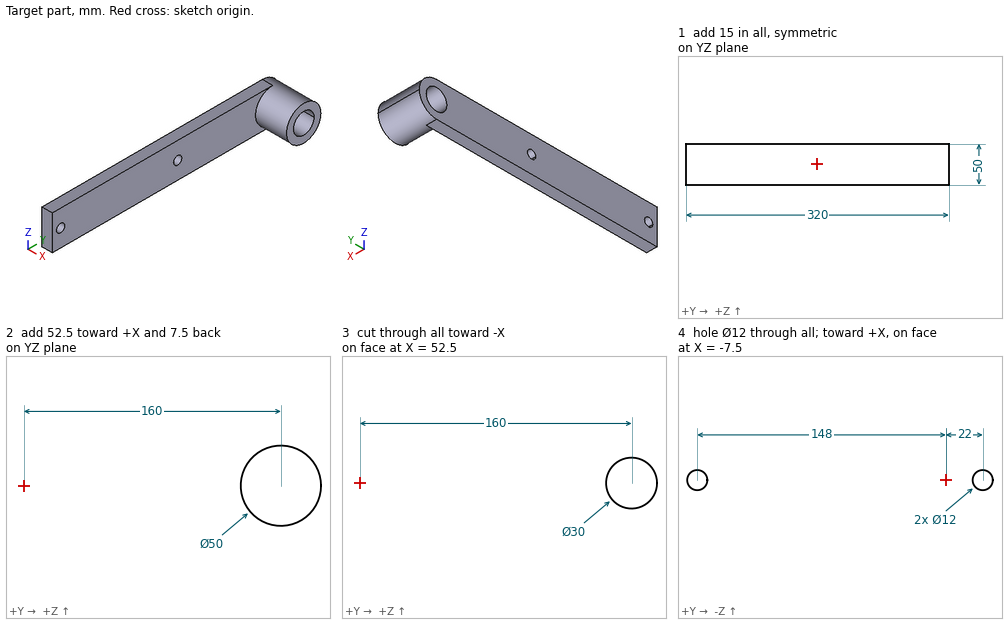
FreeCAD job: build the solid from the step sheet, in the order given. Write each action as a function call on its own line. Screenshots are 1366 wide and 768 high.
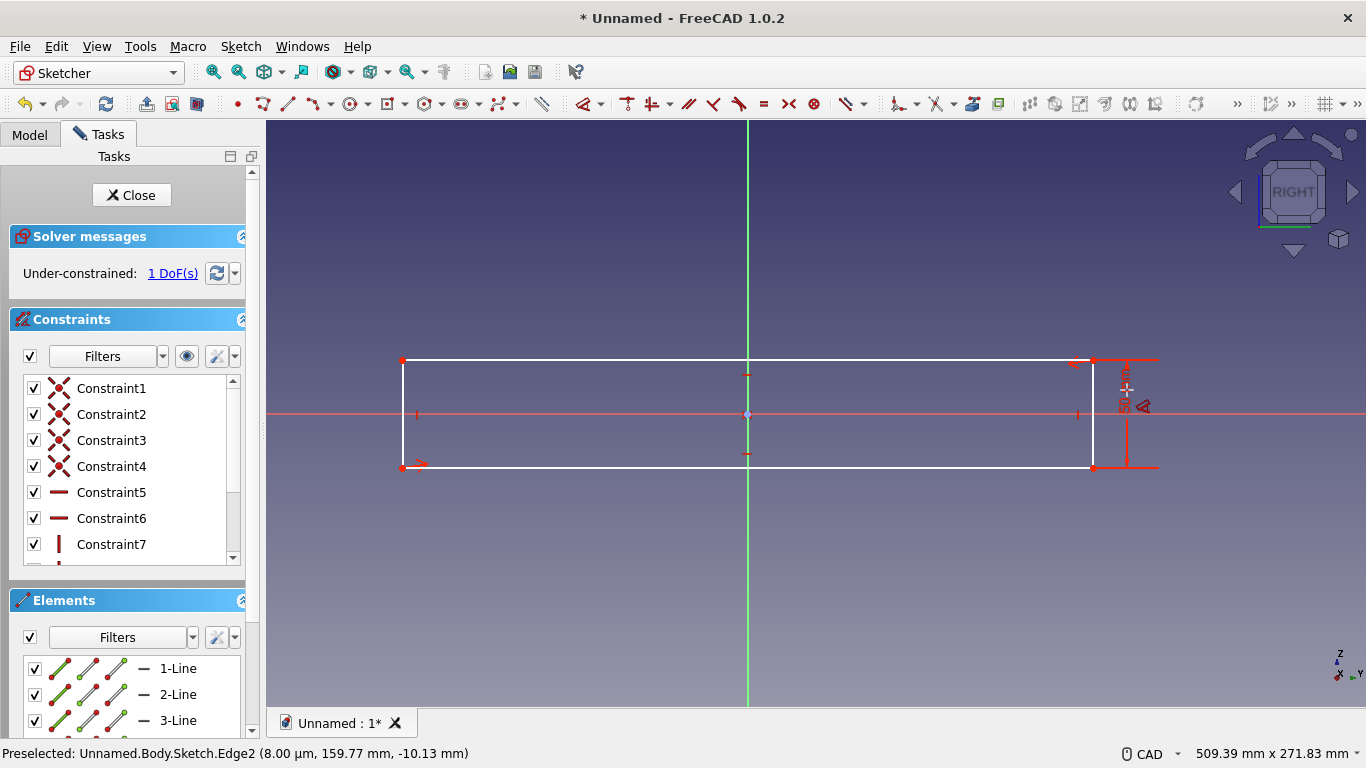
click(610, 468)
click(589, 502)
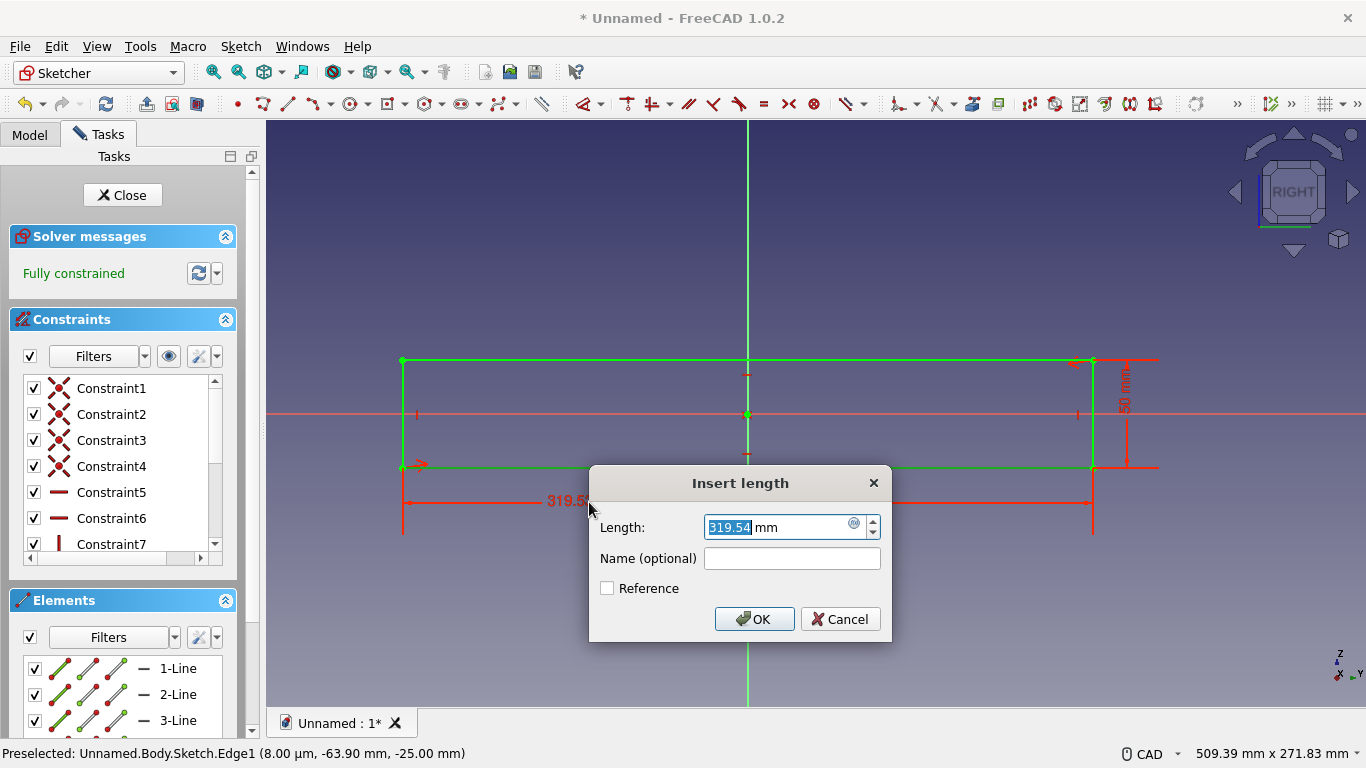
text(320)
key(Return)
key(Escape)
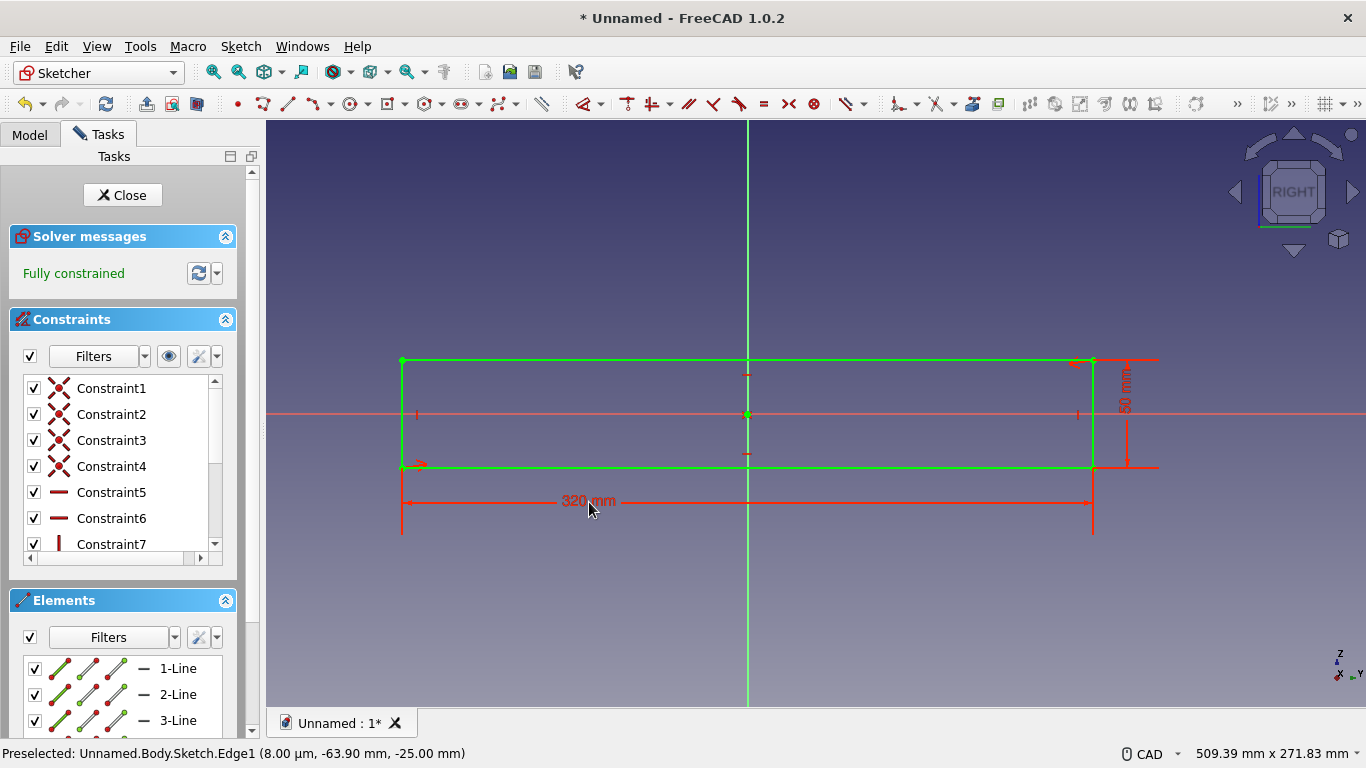
click(123, 195)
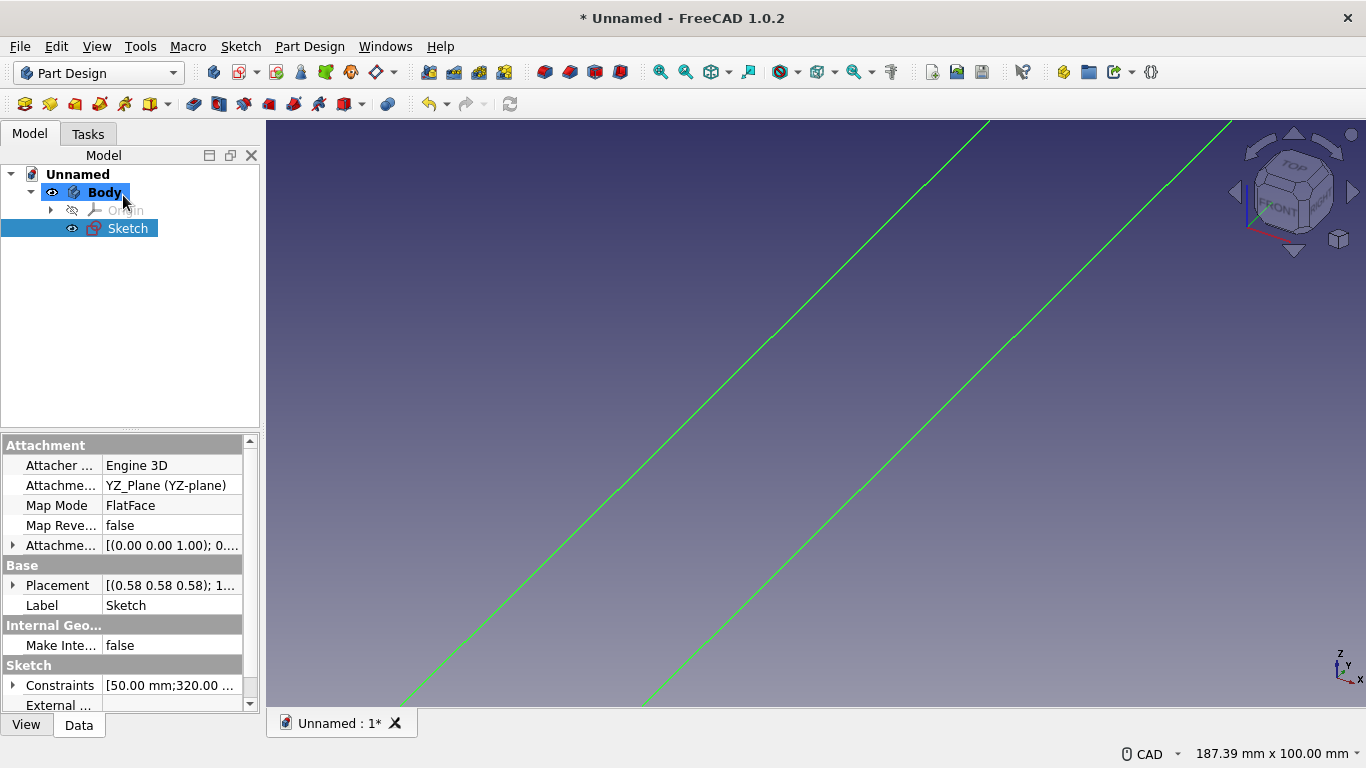
click(25, 104)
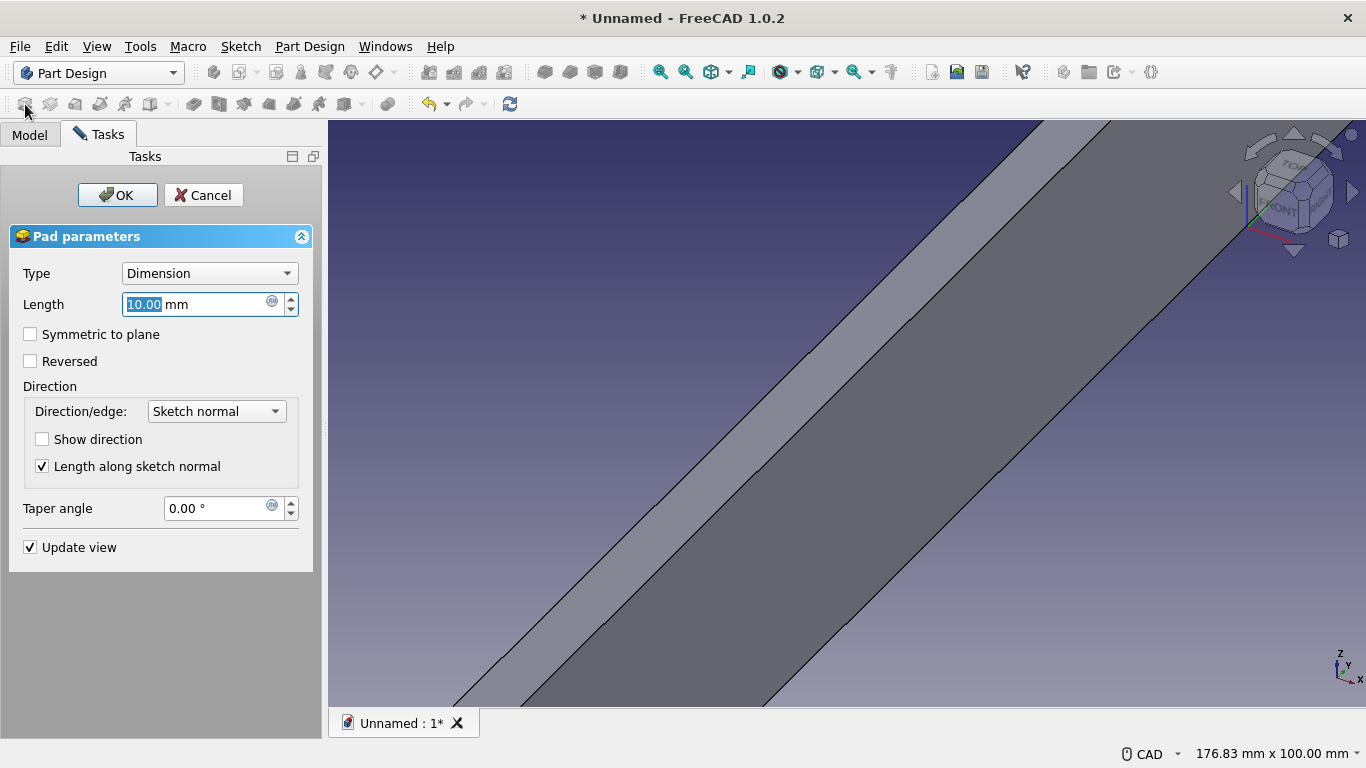
text(15)
key(Tab)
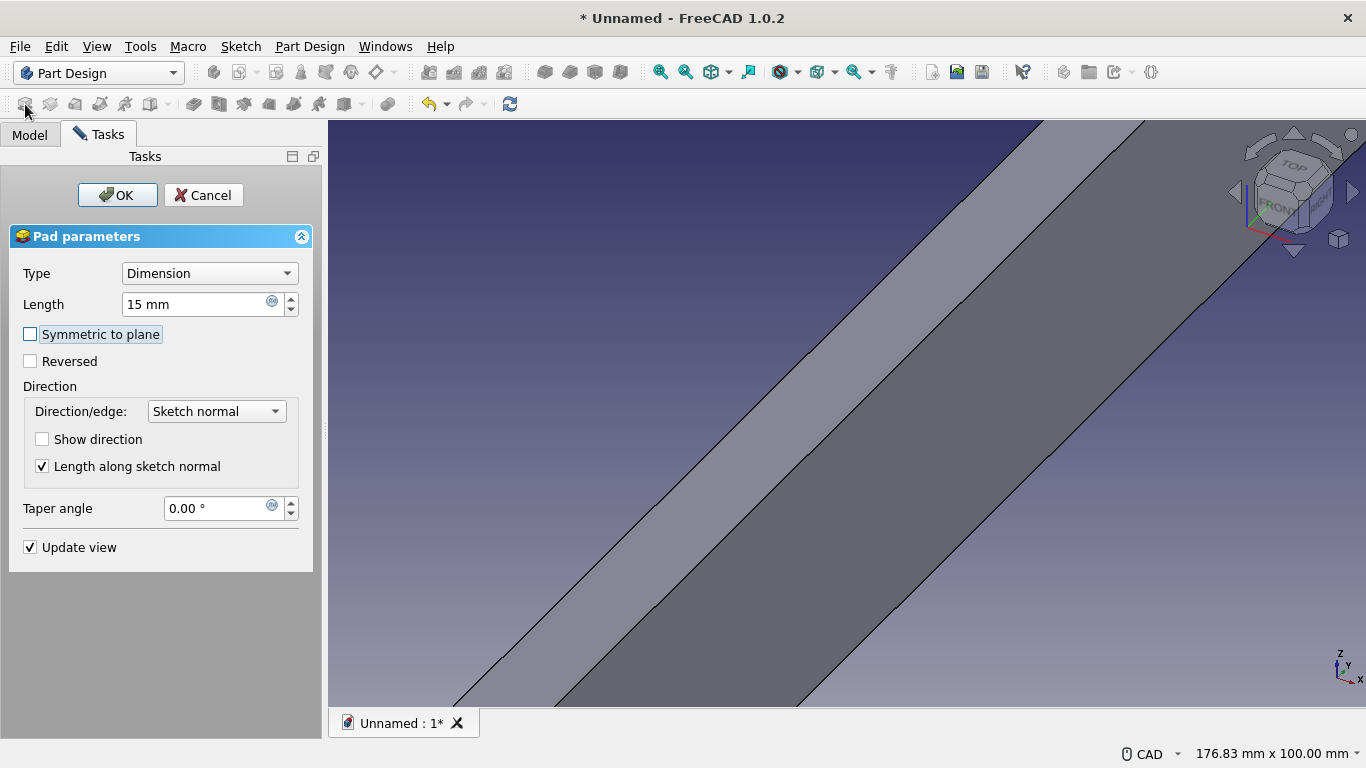
click(31, 334)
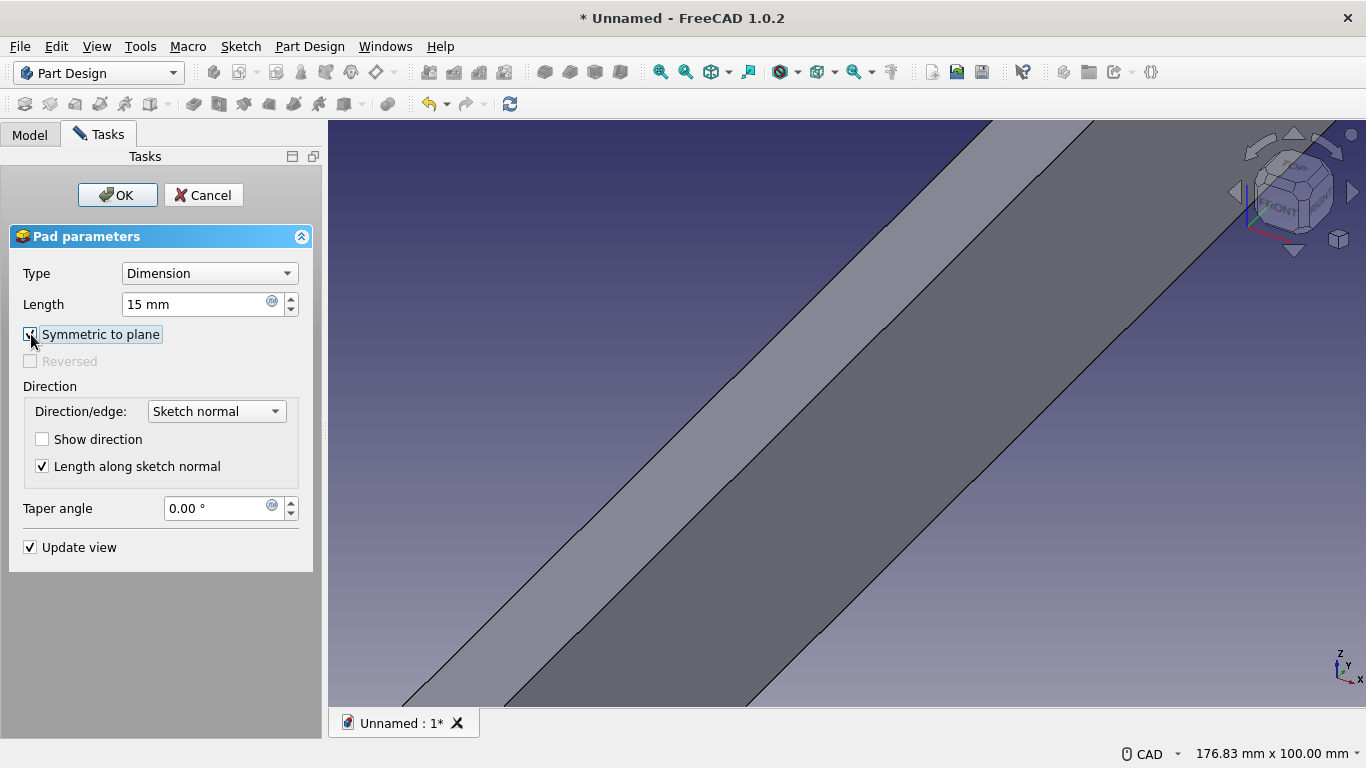
click(118, 195)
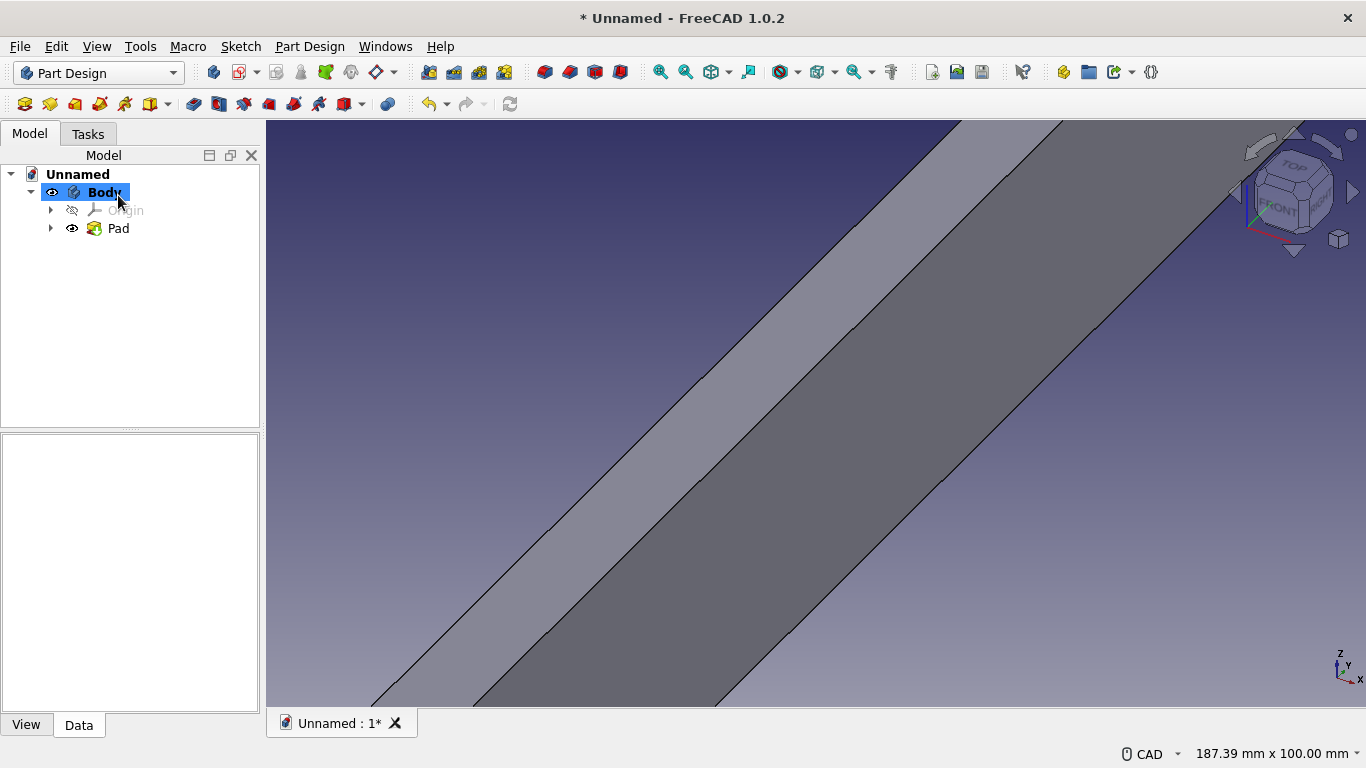
click(661, 72)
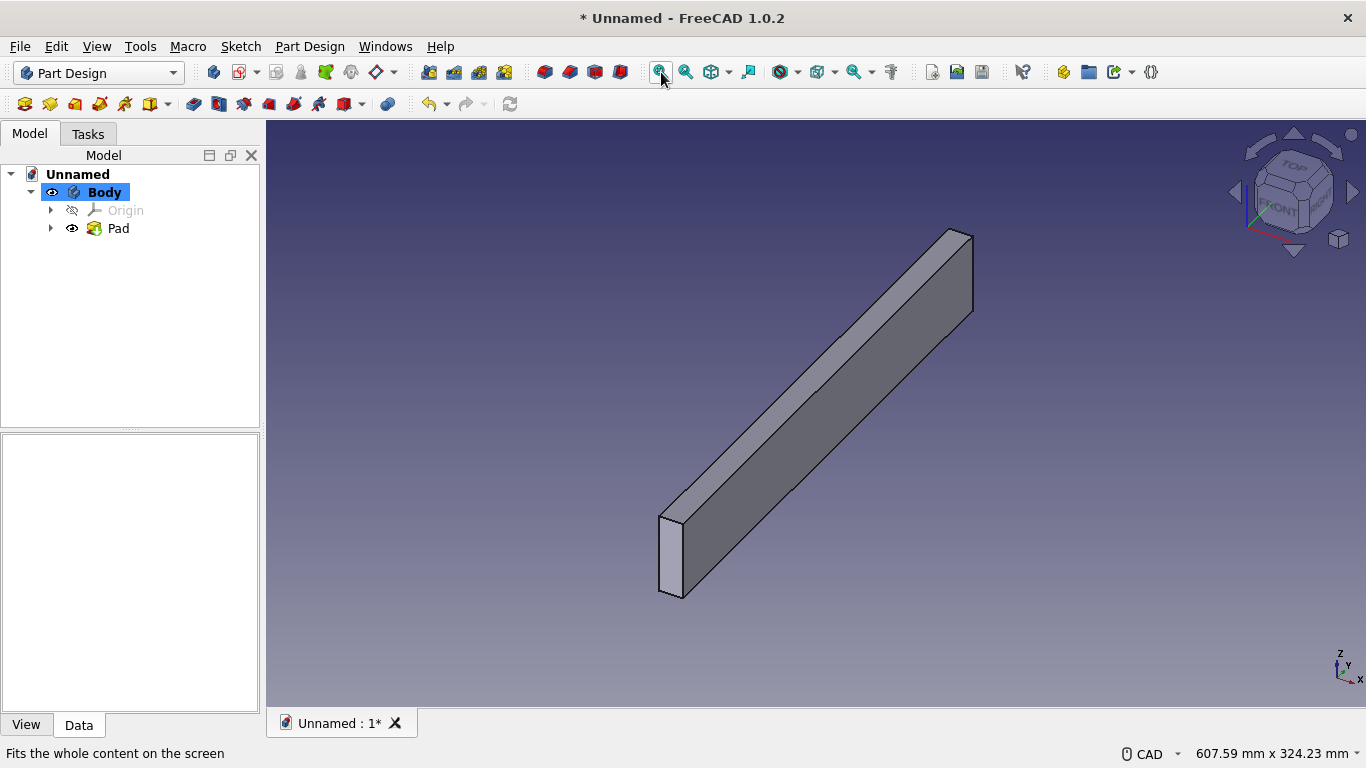
click(238, 72)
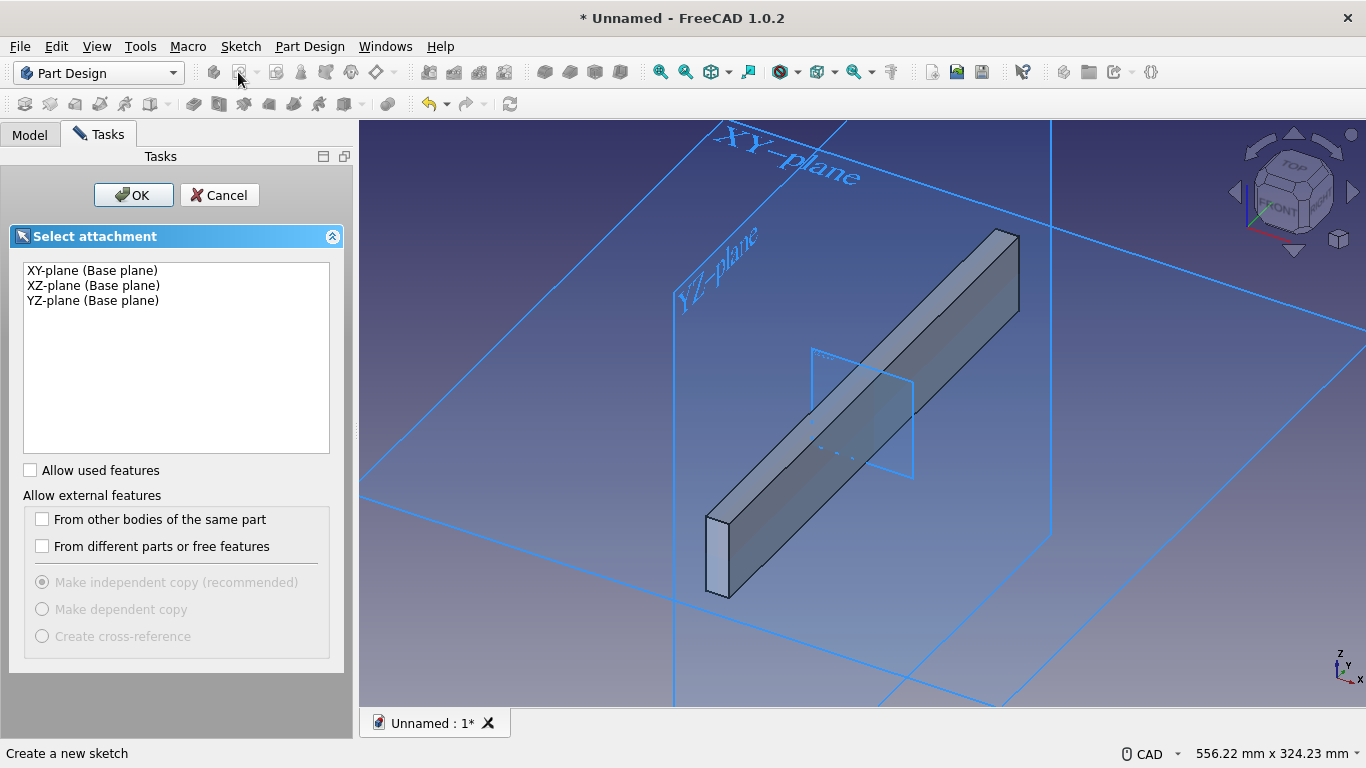
click(84, 300)